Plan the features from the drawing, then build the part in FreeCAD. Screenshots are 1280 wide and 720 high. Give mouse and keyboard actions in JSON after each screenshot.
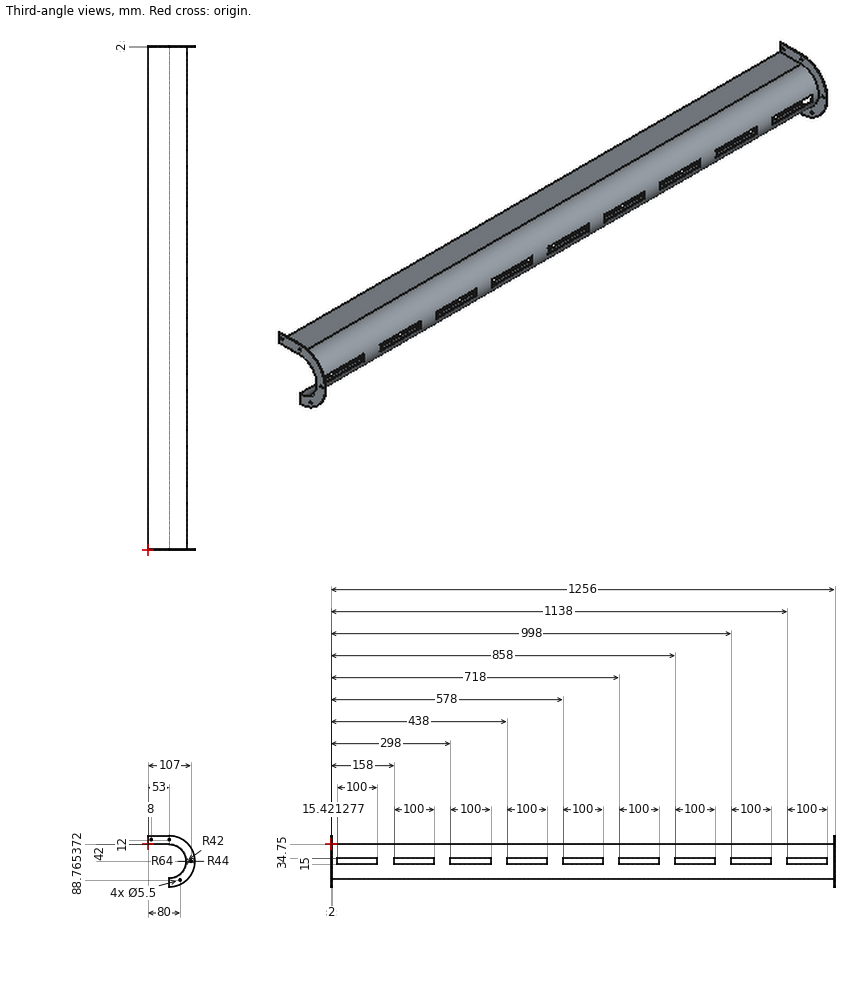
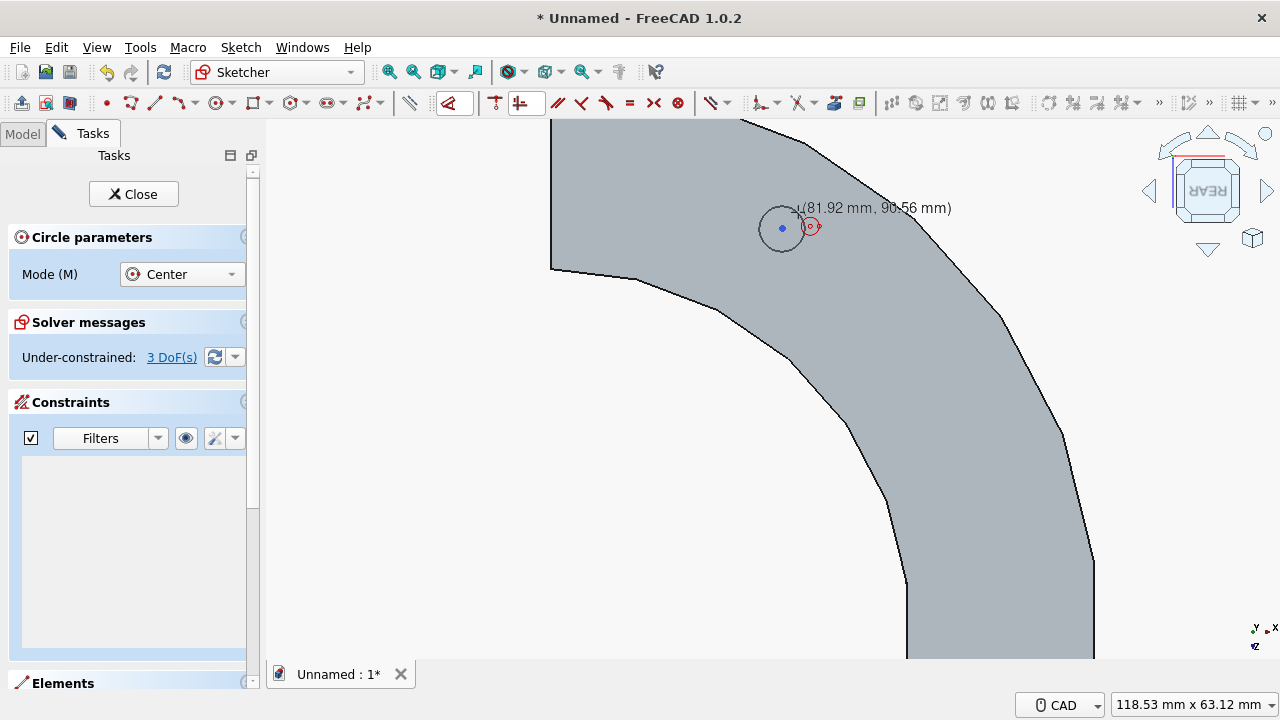
{"action": "left_click", "coordinate": [1013, 628]}
{"action": "left_click", "coordinate": [1029, 612]}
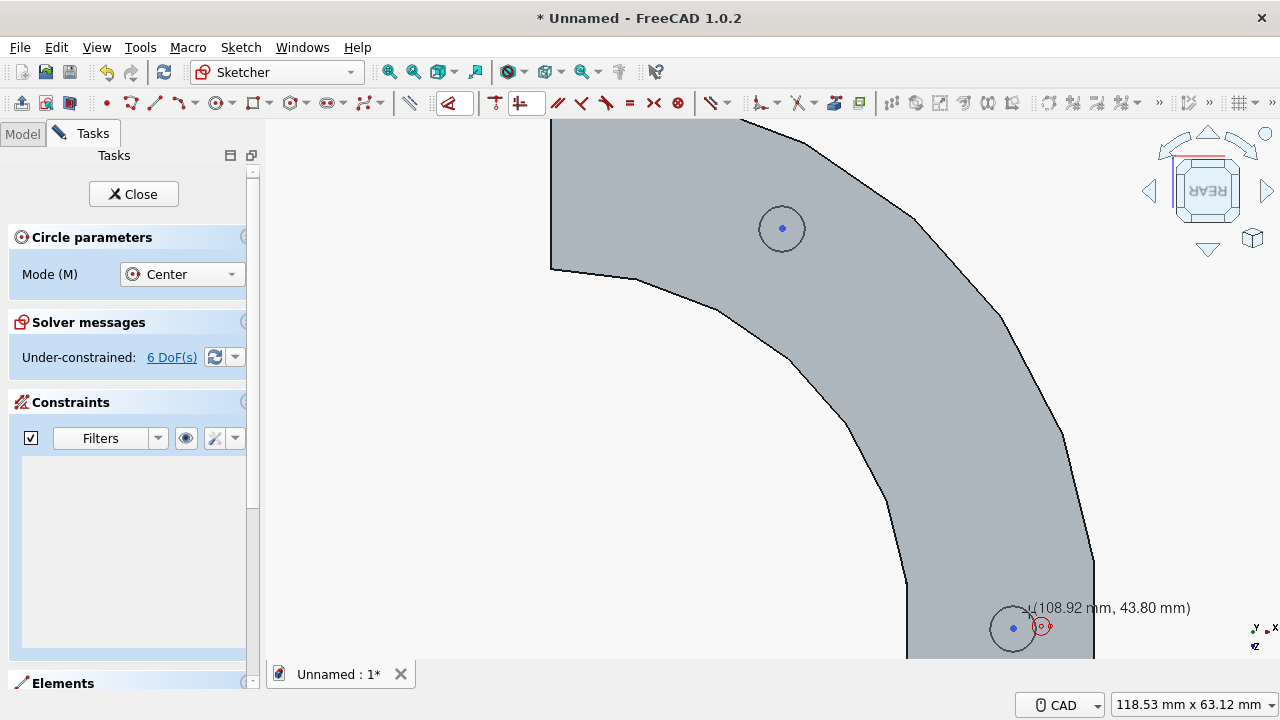
{"action": "scroll", "coordinate": [785, 232], "scroll_direction": "down", "scroll_amount": 5}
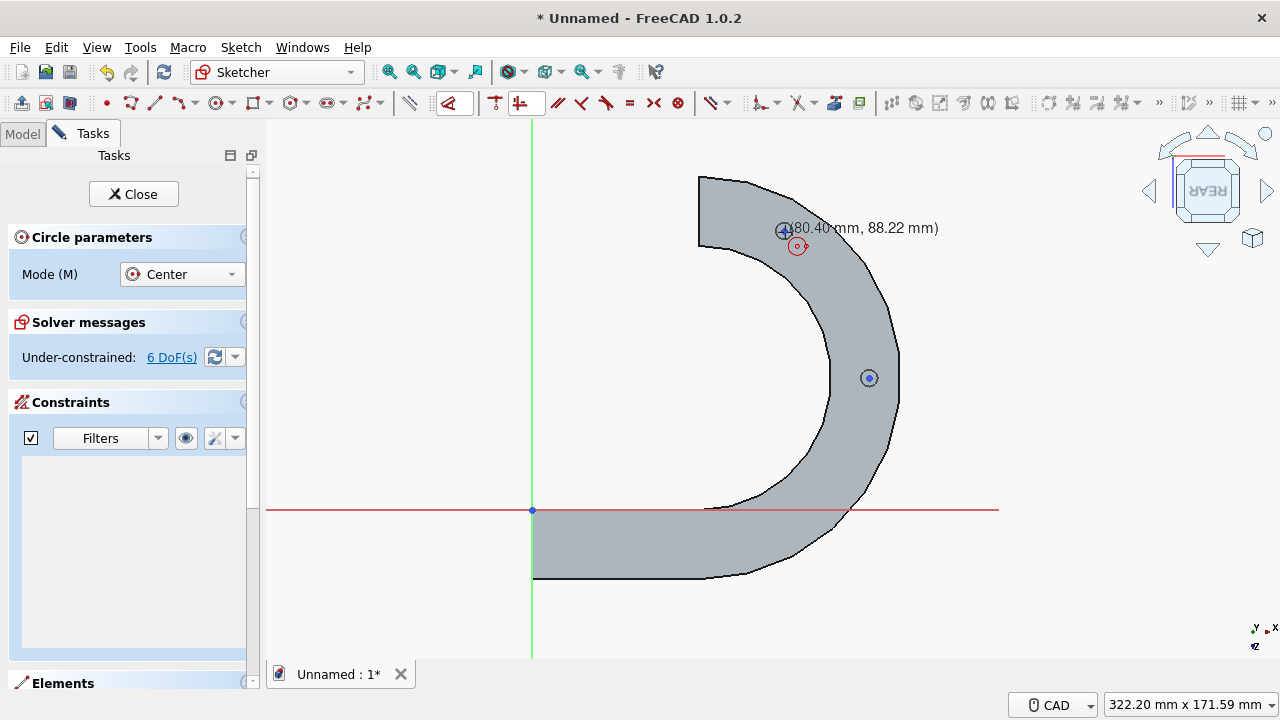
{"action": "scroll", "coordinate": [699, 548], "scroll_direction": "up", "scroll_amount": 5}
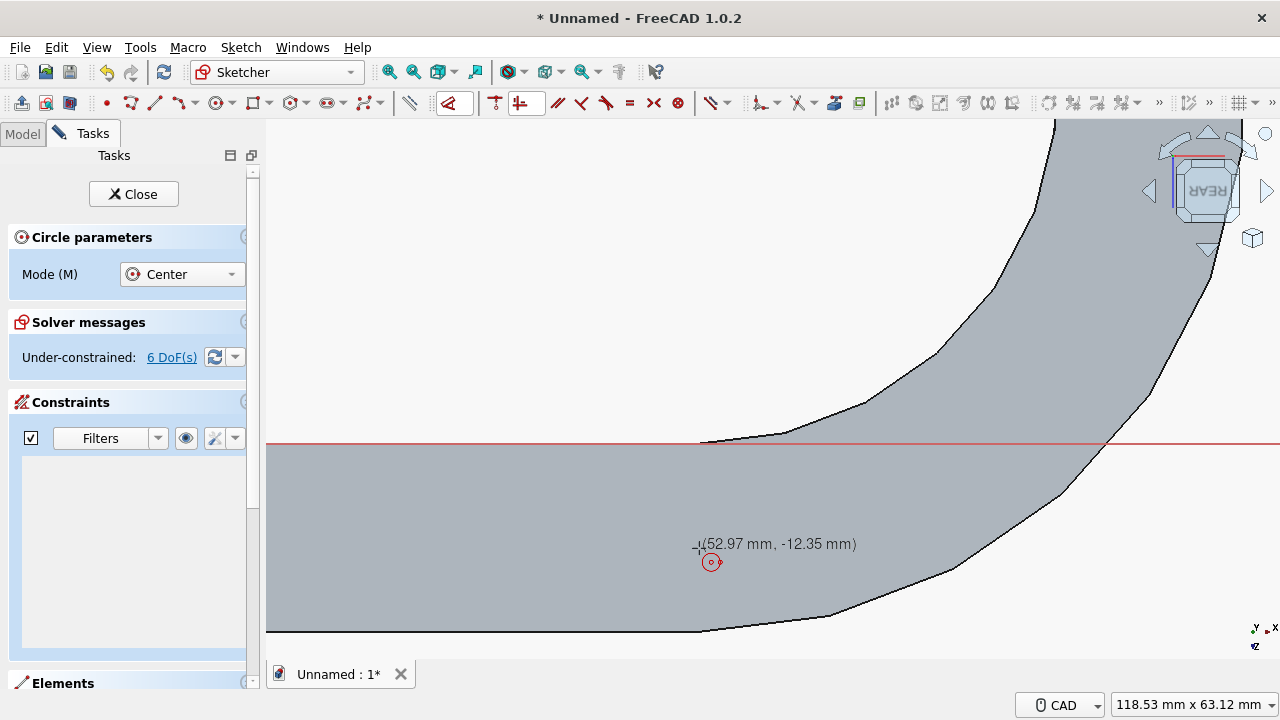
{"action": "left_click", "coordinate": [699, 546]}
{"action": "left_click", "coordinate": [715, 530]}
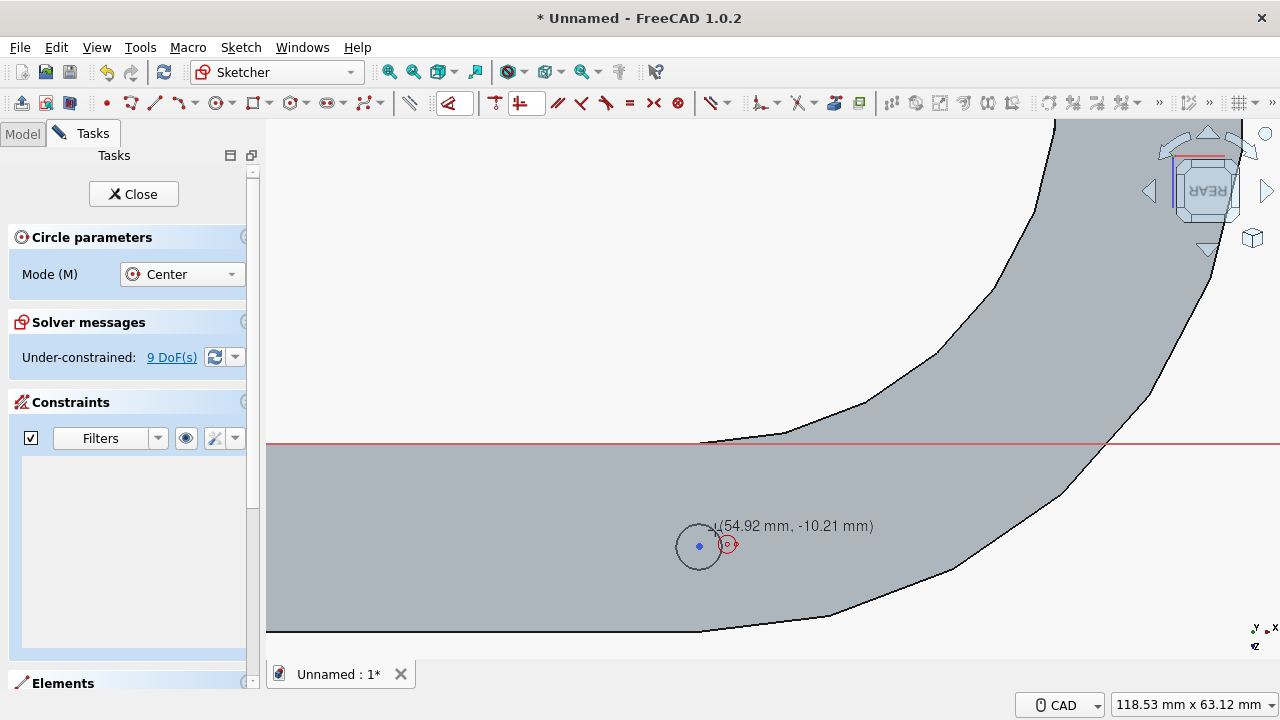
{"action": "left_click", "coordinate": [314, 546]}
{"action": "left_click", "coordinate": [330, 530]}
{"action": "key", "text": "Escape"}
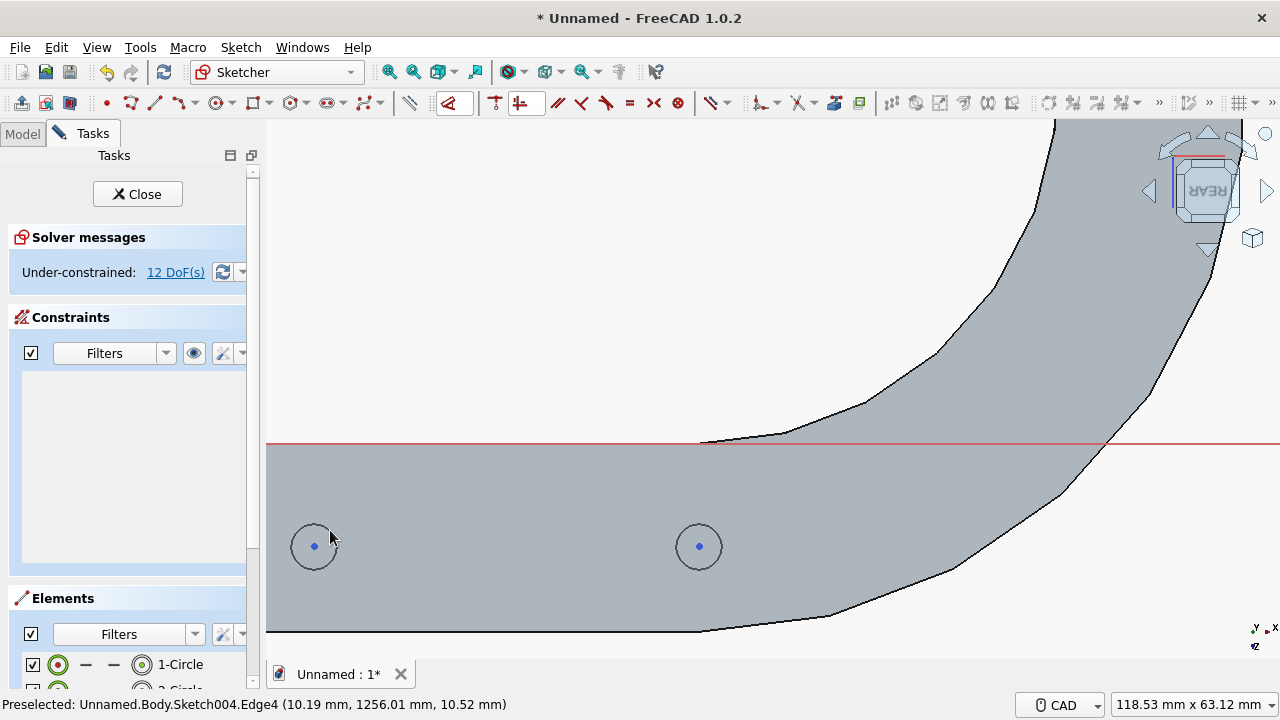
{"action": "scroll", "coordinate": [699, 548], "scroll_direction": "down", "scroll_amount": 5}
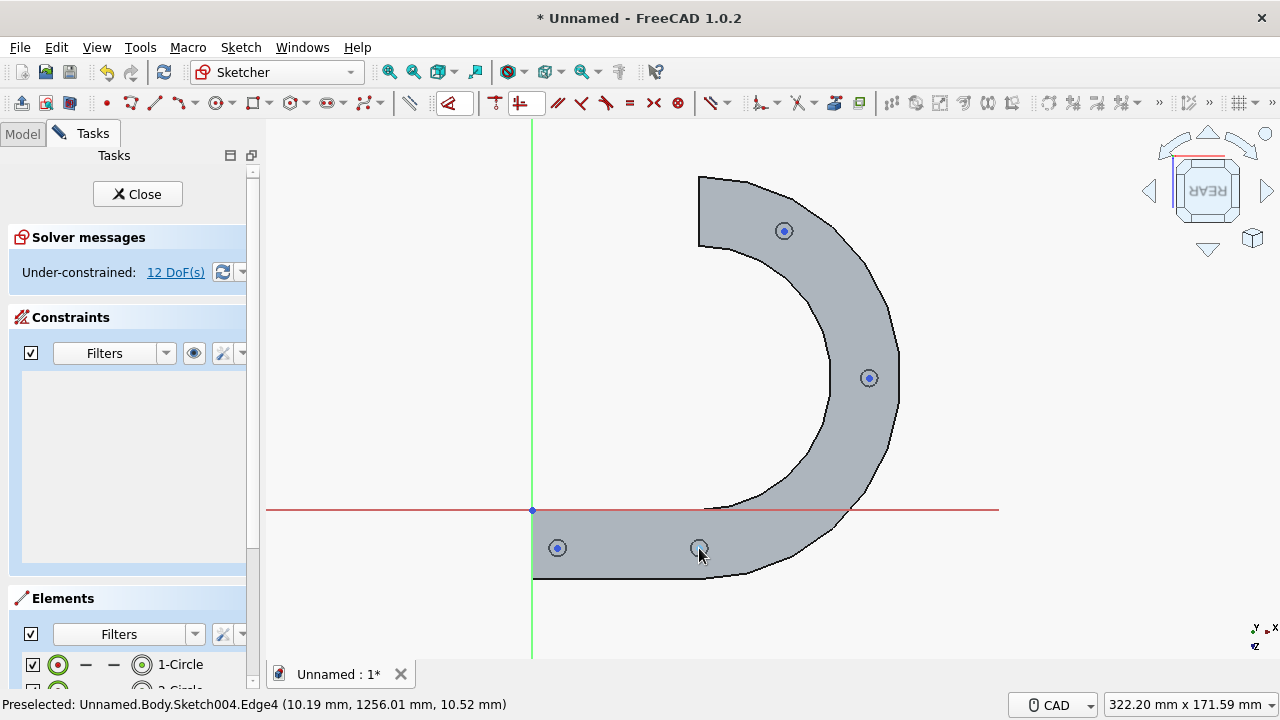
{"action": "scroll", "coordinate": [790, 225], "scroll_direction": "up", "scroll_amount": 3}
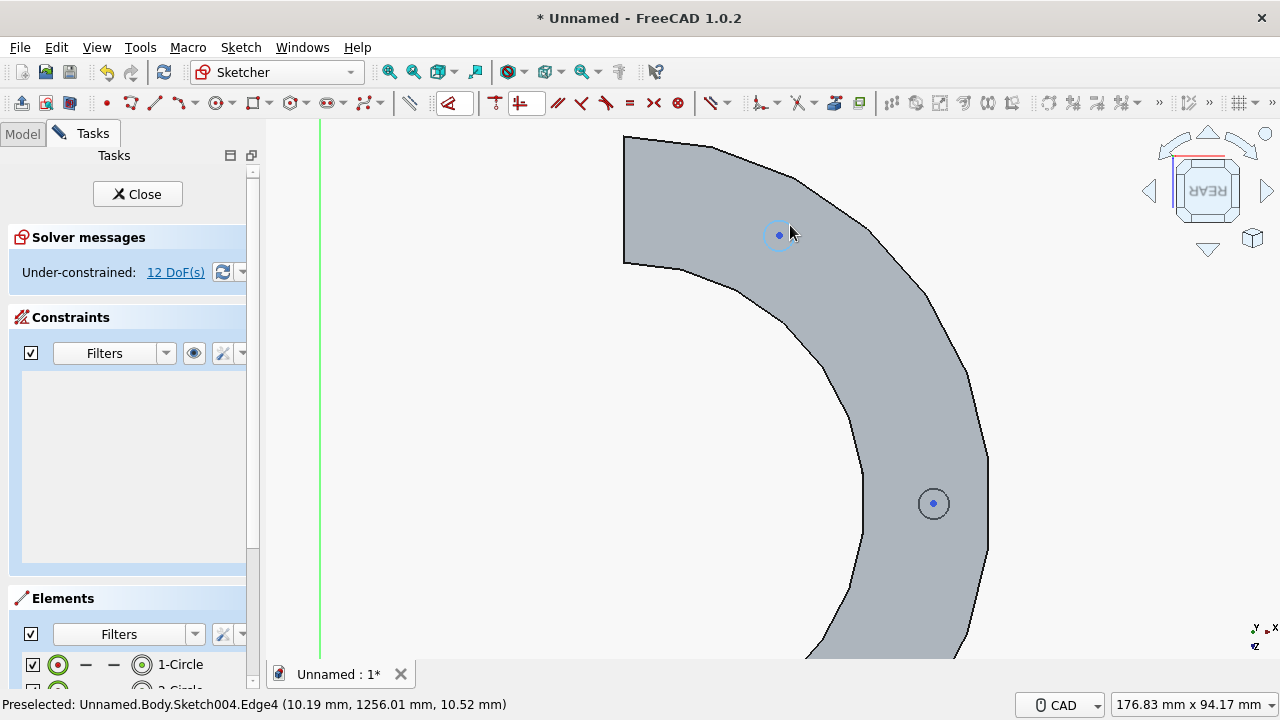
{"action": "left_click", "coordinate": [790, 225]}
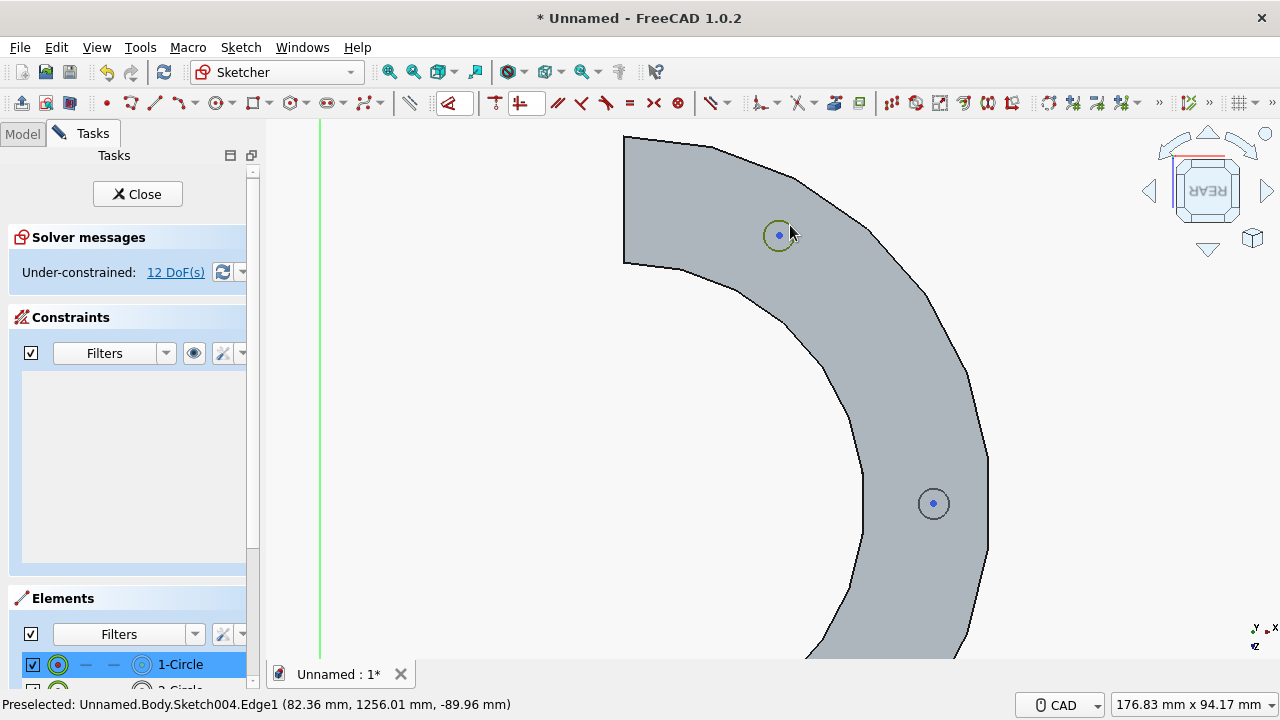
{"action": "left_click", "coordinate": [945, 493]}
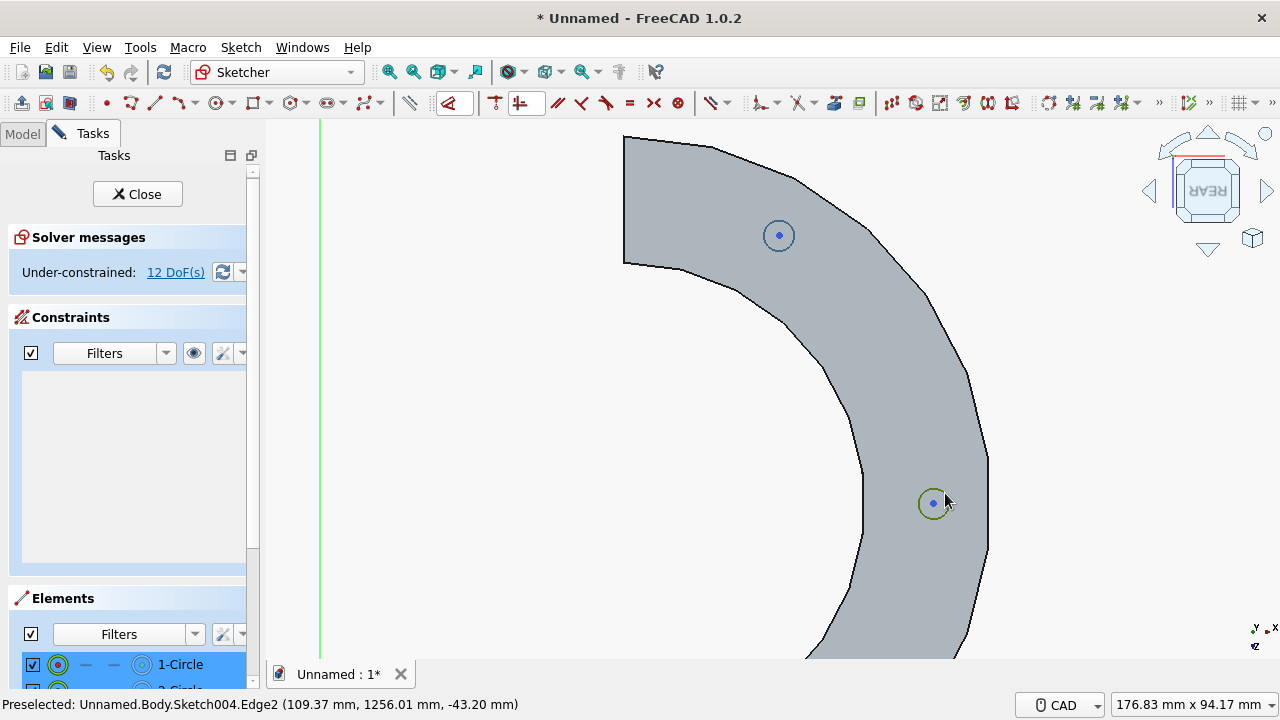
{"action": "scroll", "coordinate": [789, 224], "scroll_direction": "down", "scroll_amount": 3}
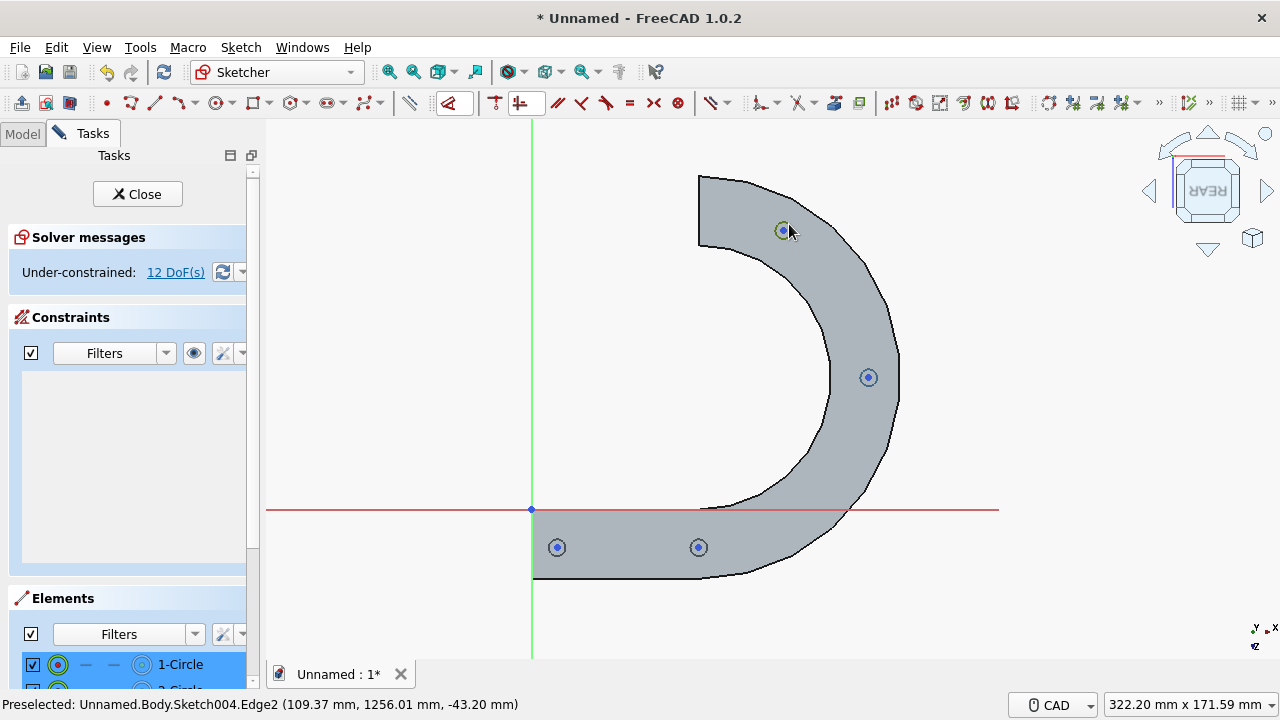
{"action": "scroll", "coordinate": [705, 542], "scroll_direction": "up", "scroll_amount": 3}